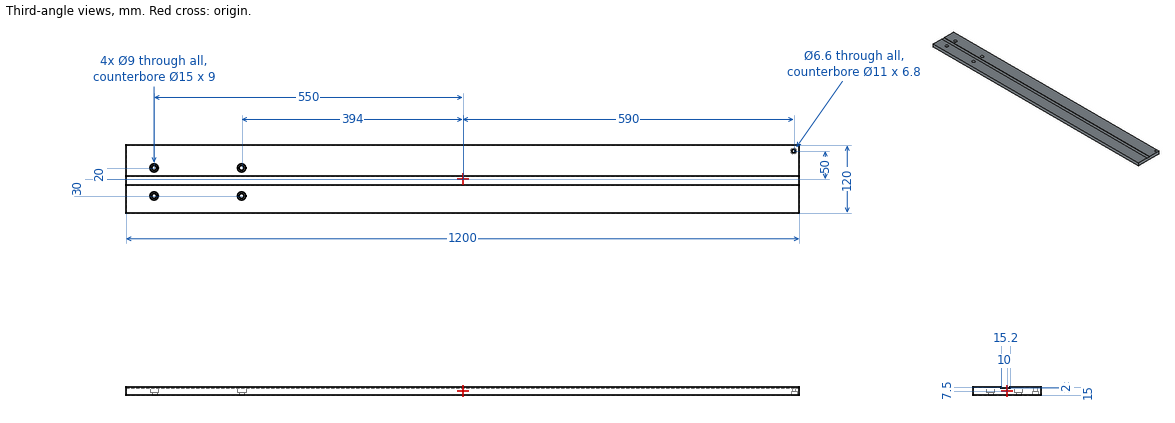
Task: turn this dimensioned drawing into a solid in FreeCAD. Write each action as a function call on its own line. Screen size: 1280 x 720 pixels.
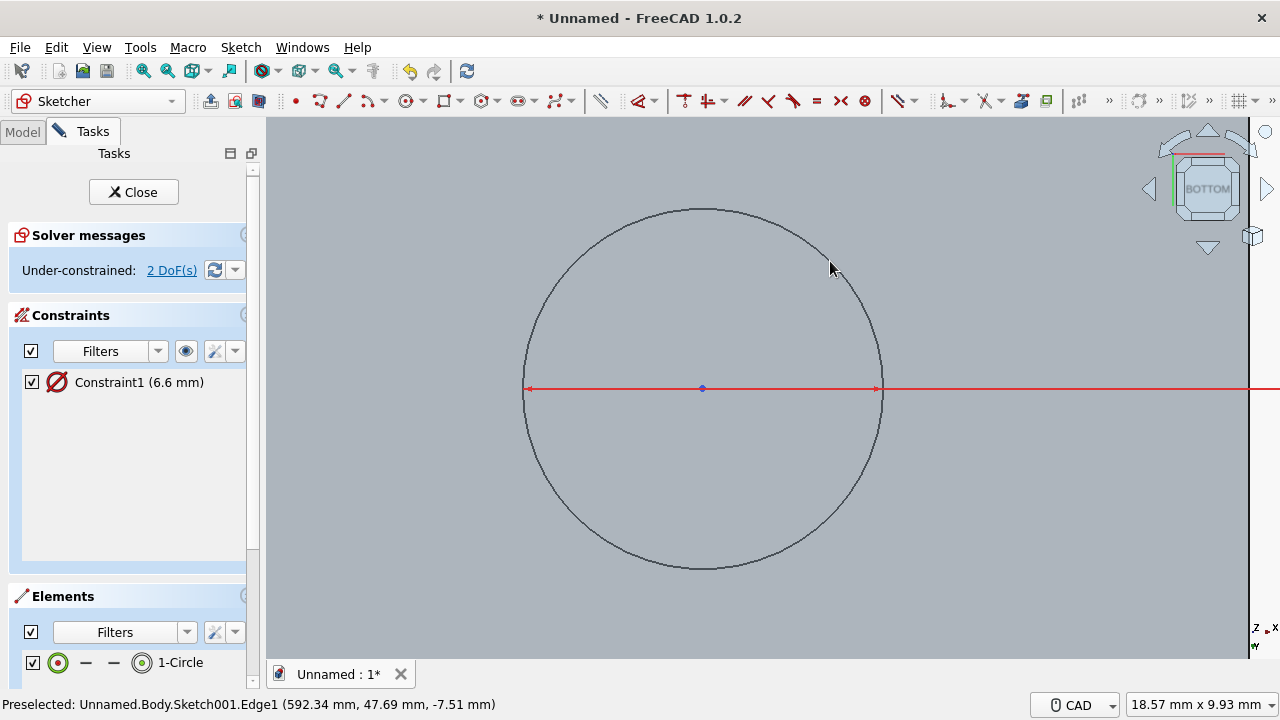
click(703, 389)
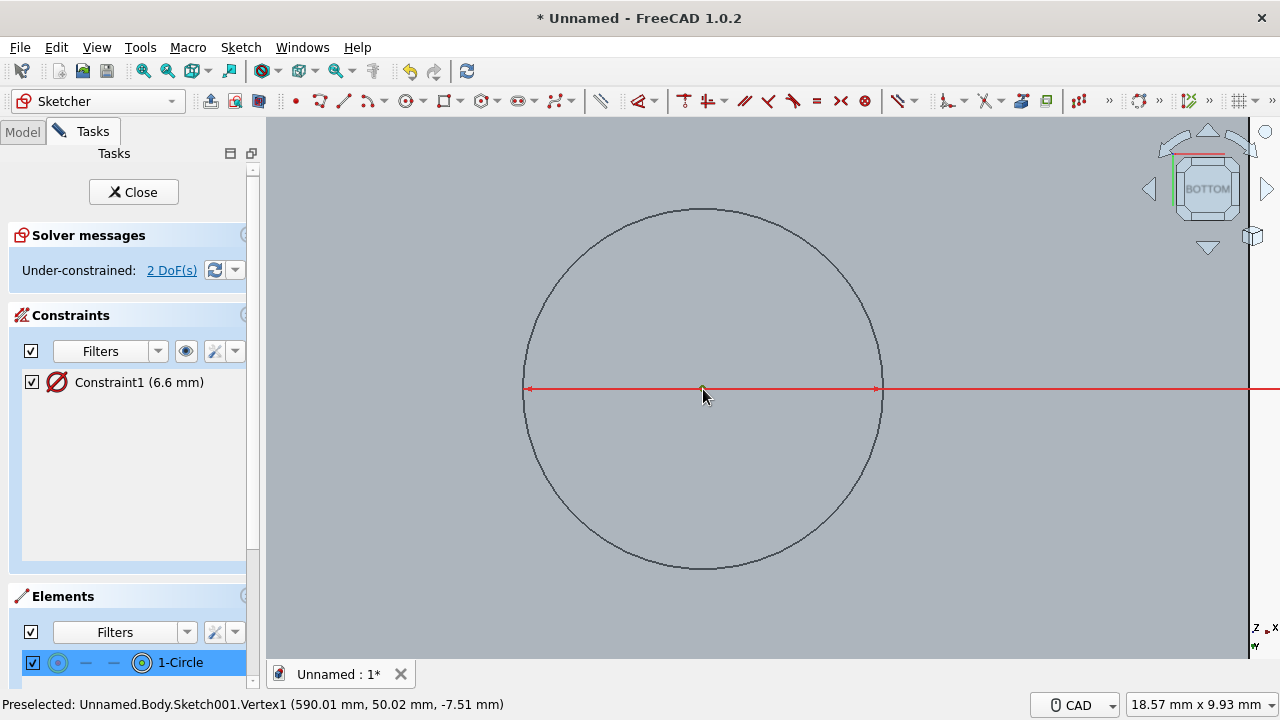
click(656, 102)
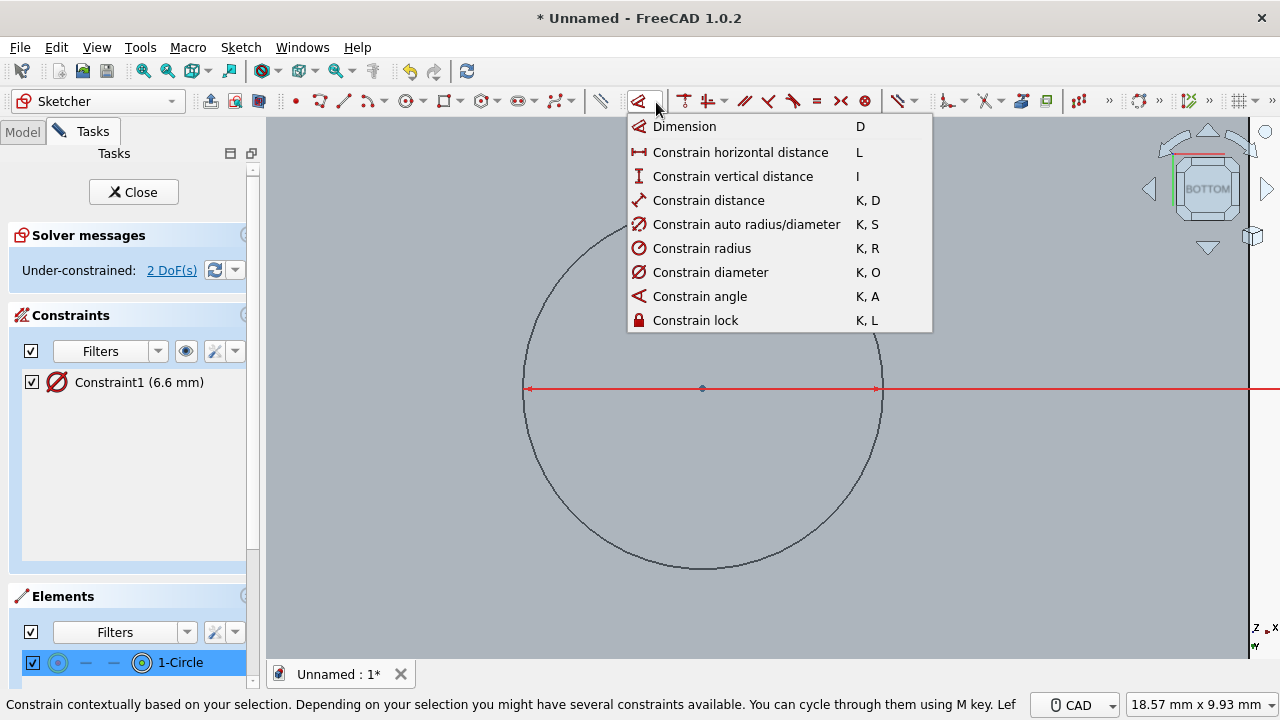
click(780, 176)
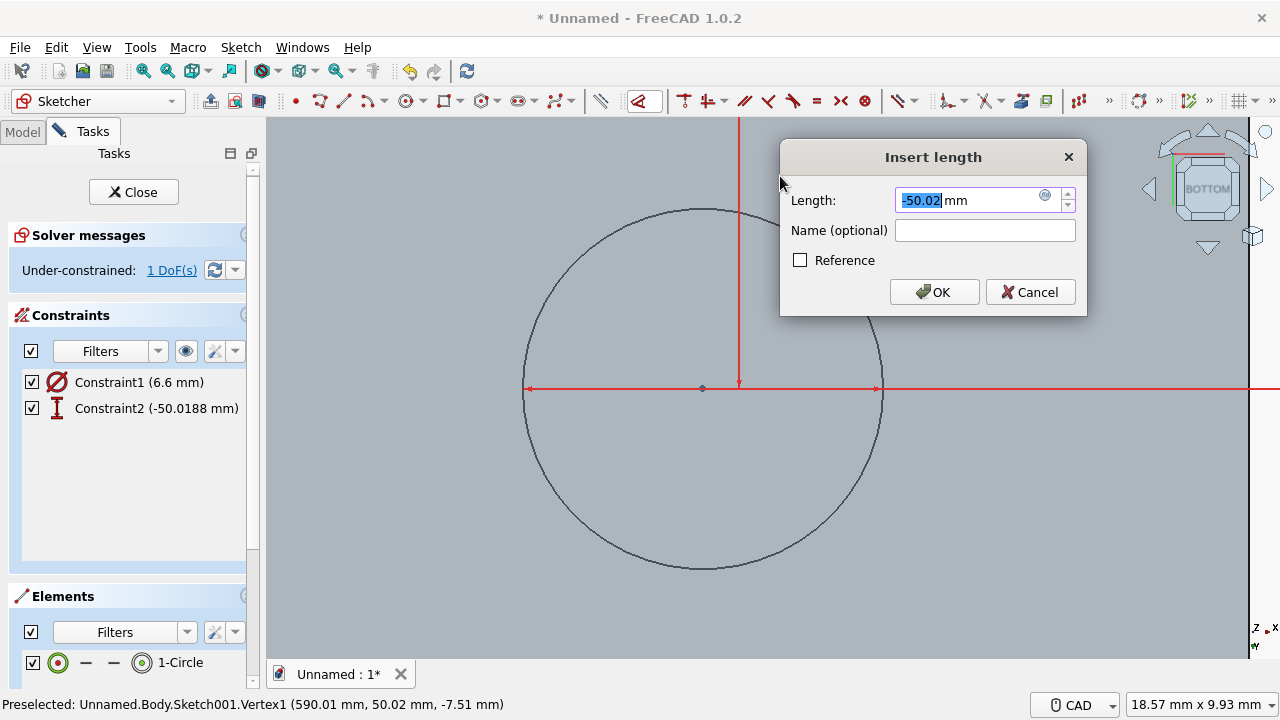
text(-50)
key(Return)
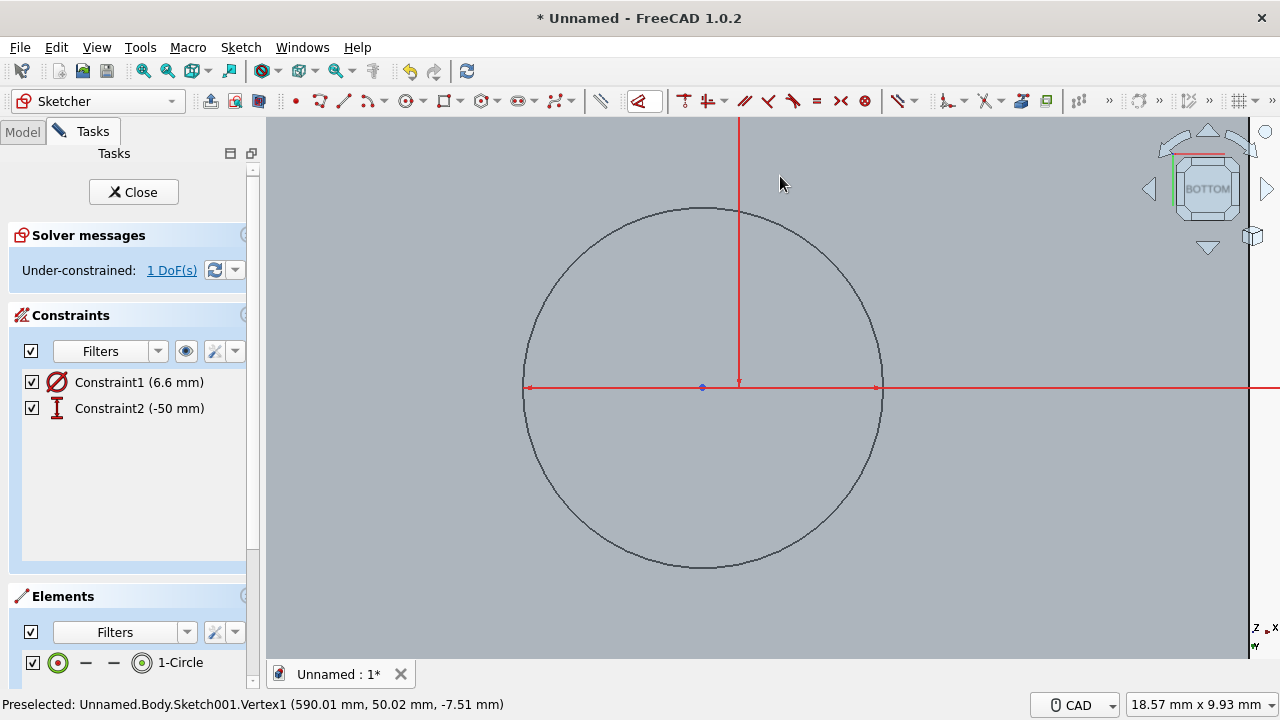
click(703, 388)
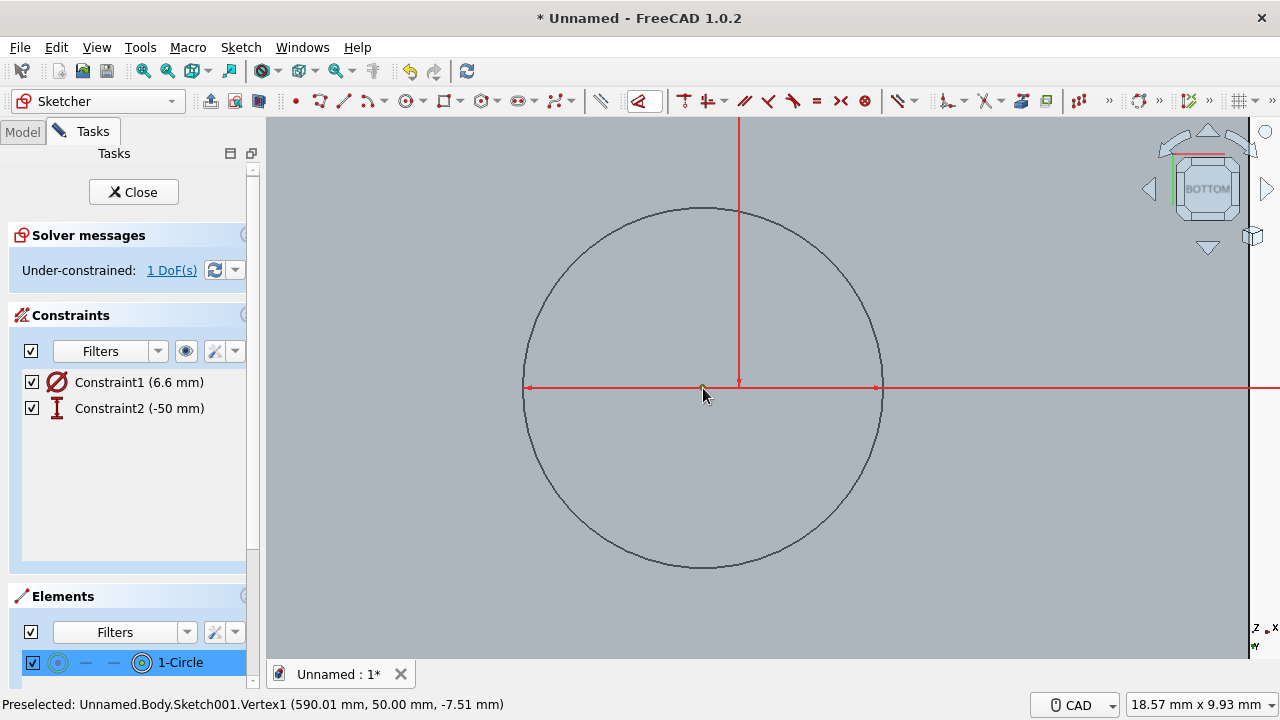
click(656, 102)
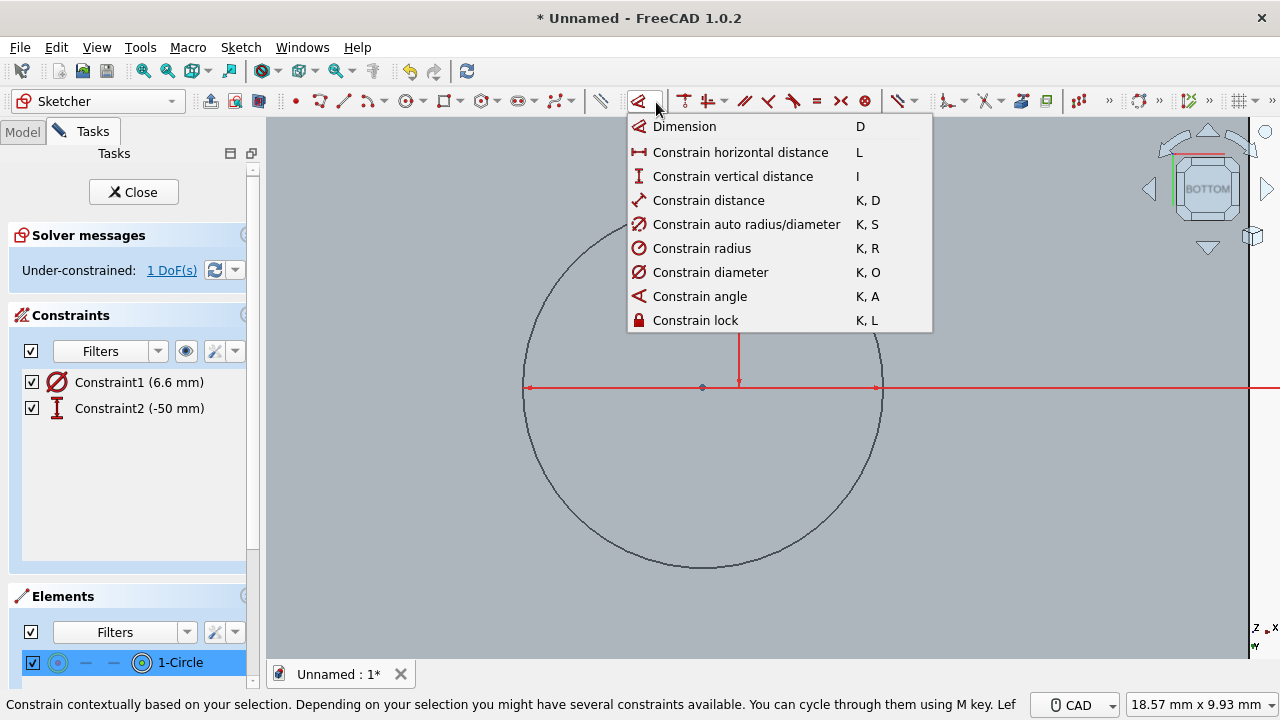
click(780, 152)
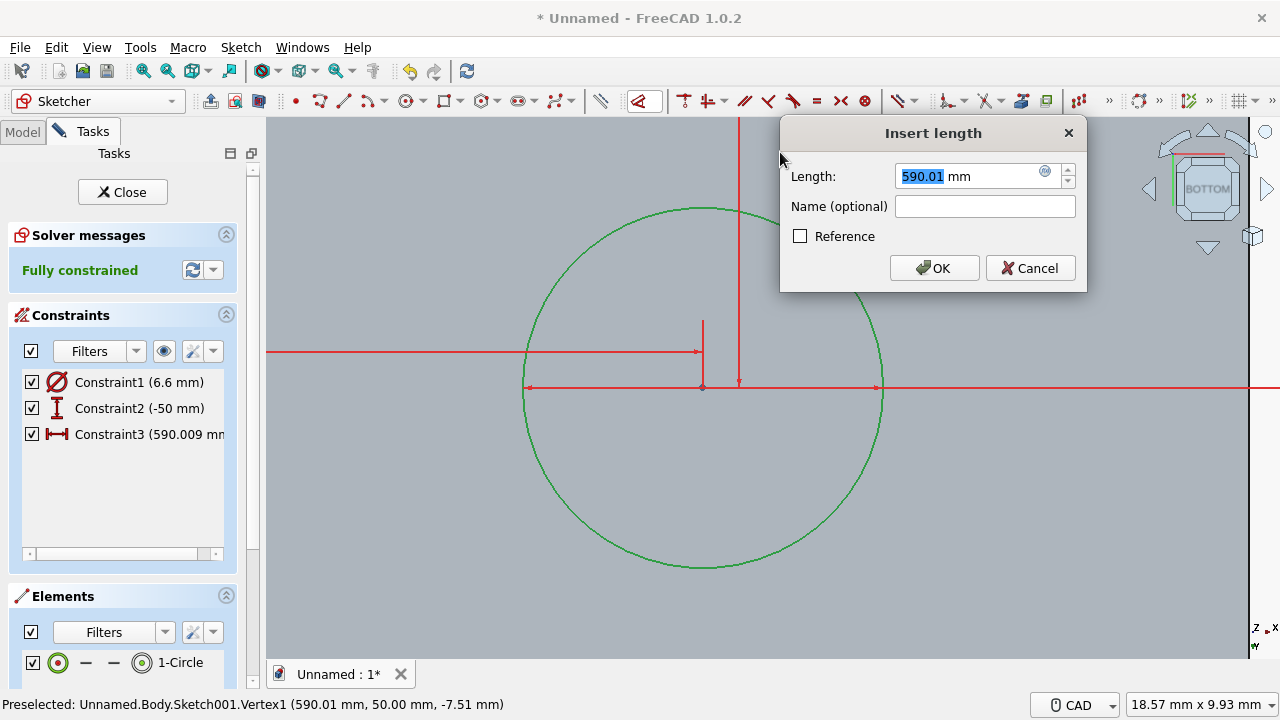
text(590)
key(Return)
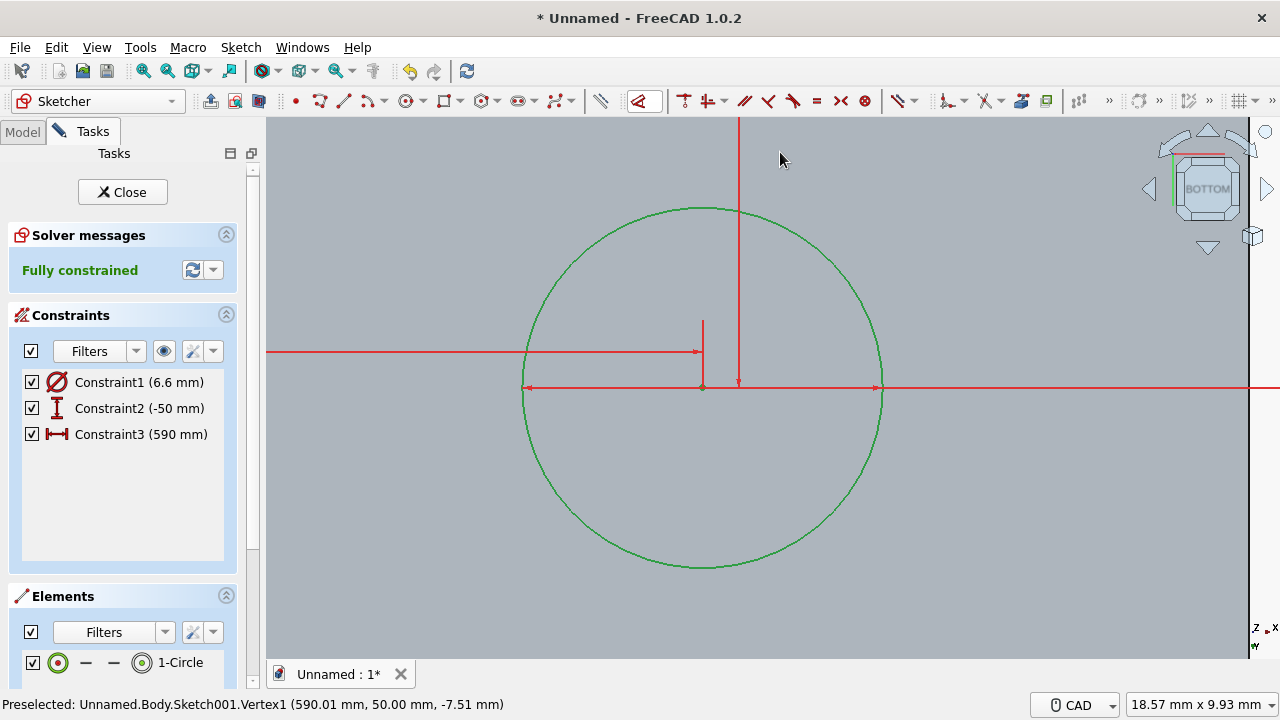
click(123, 192)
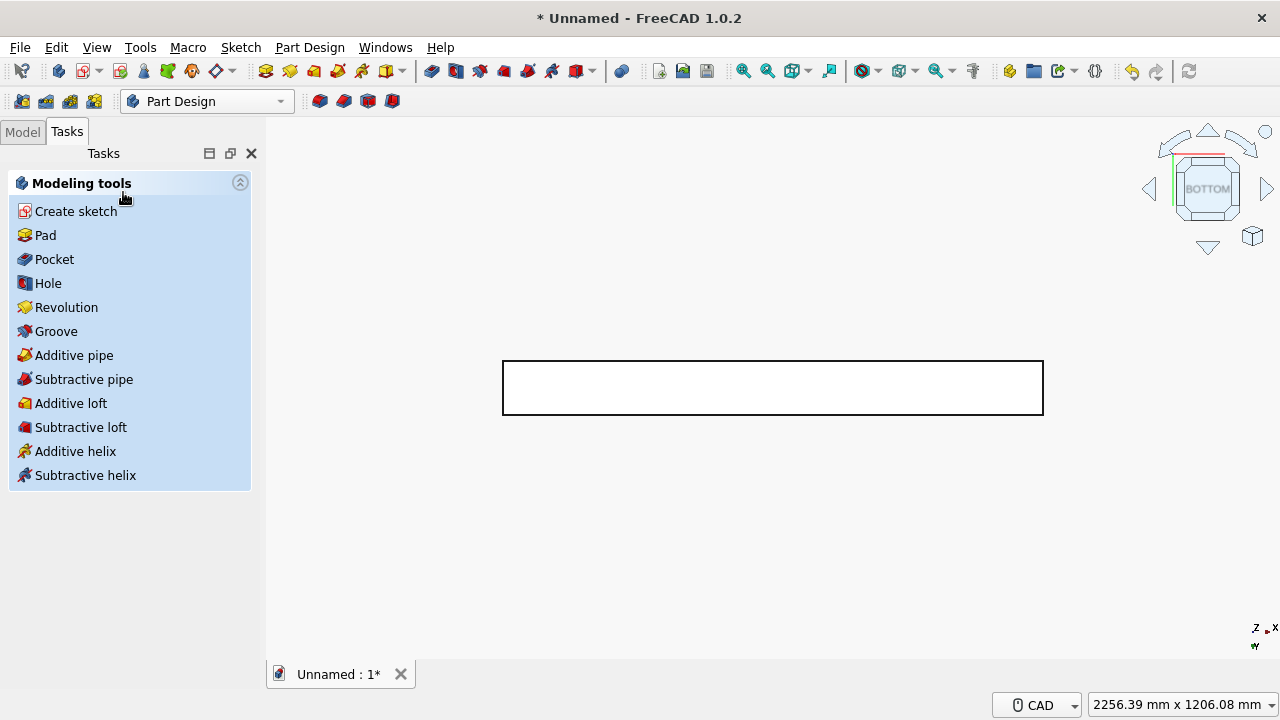
click(456, 72)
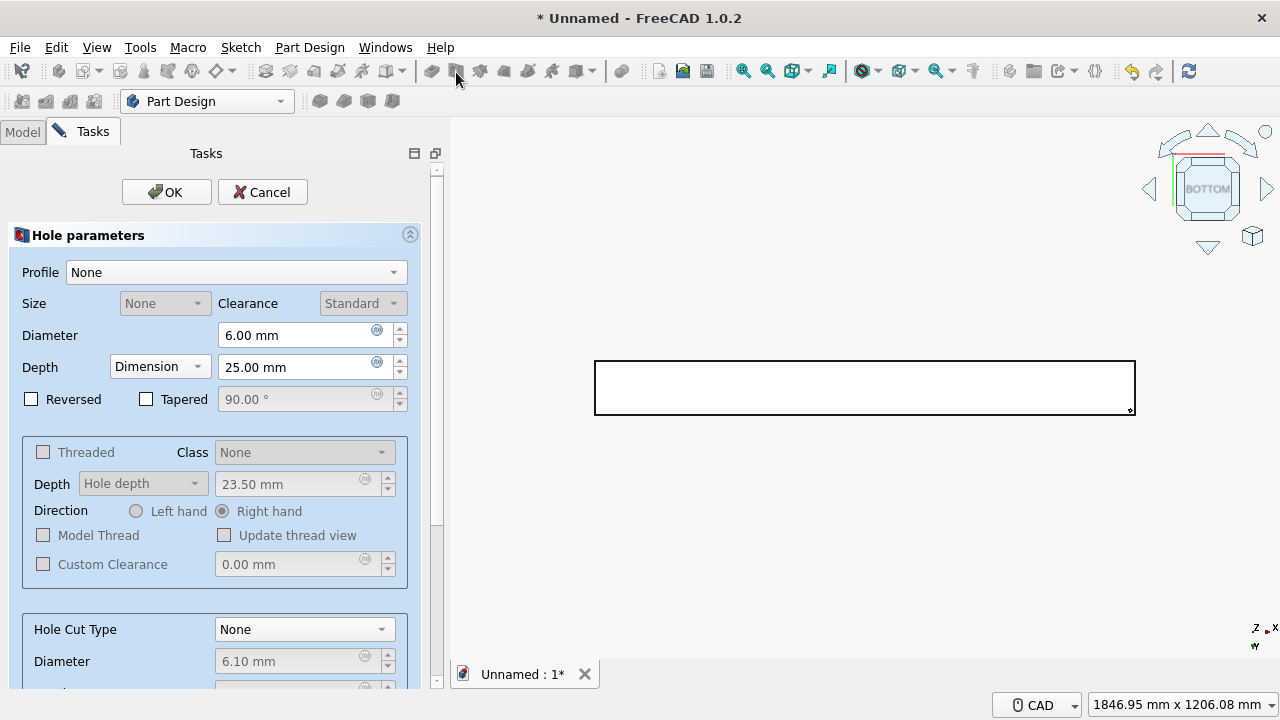
triple_click(305, 335)